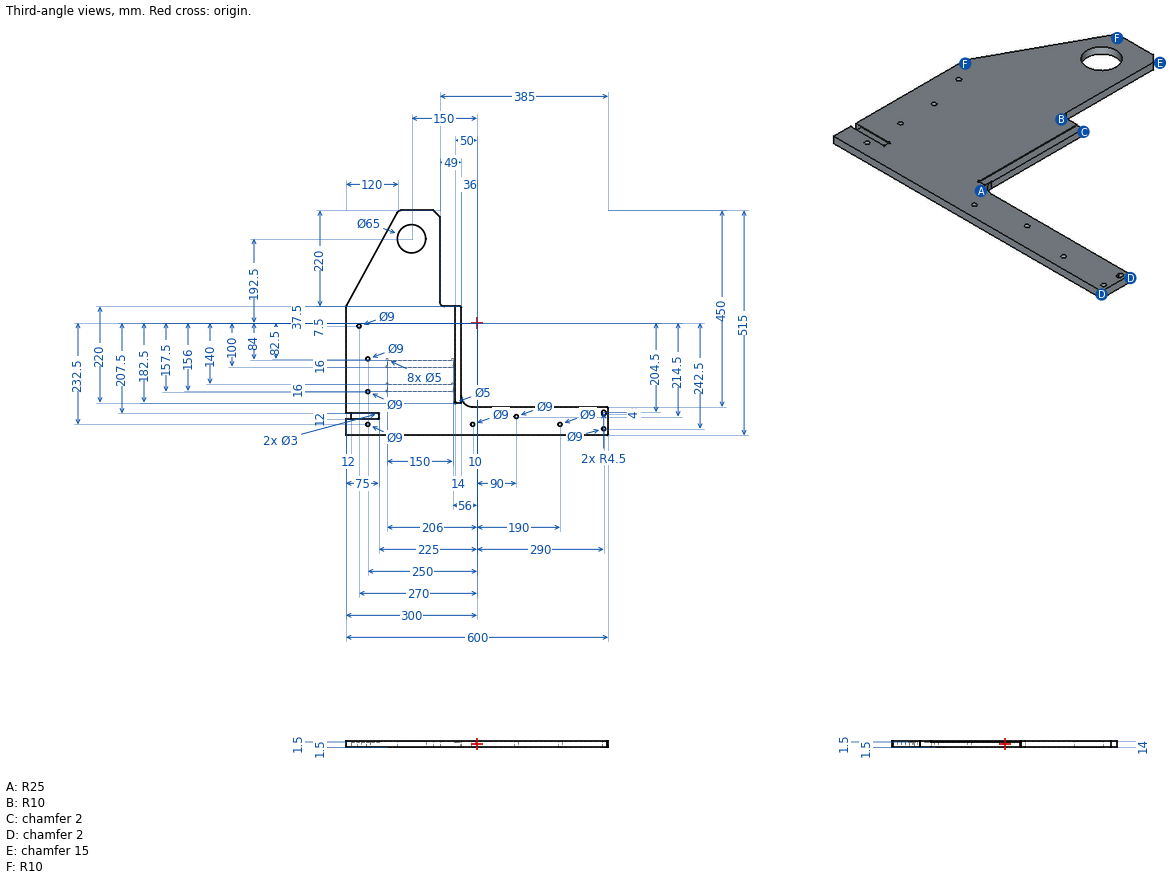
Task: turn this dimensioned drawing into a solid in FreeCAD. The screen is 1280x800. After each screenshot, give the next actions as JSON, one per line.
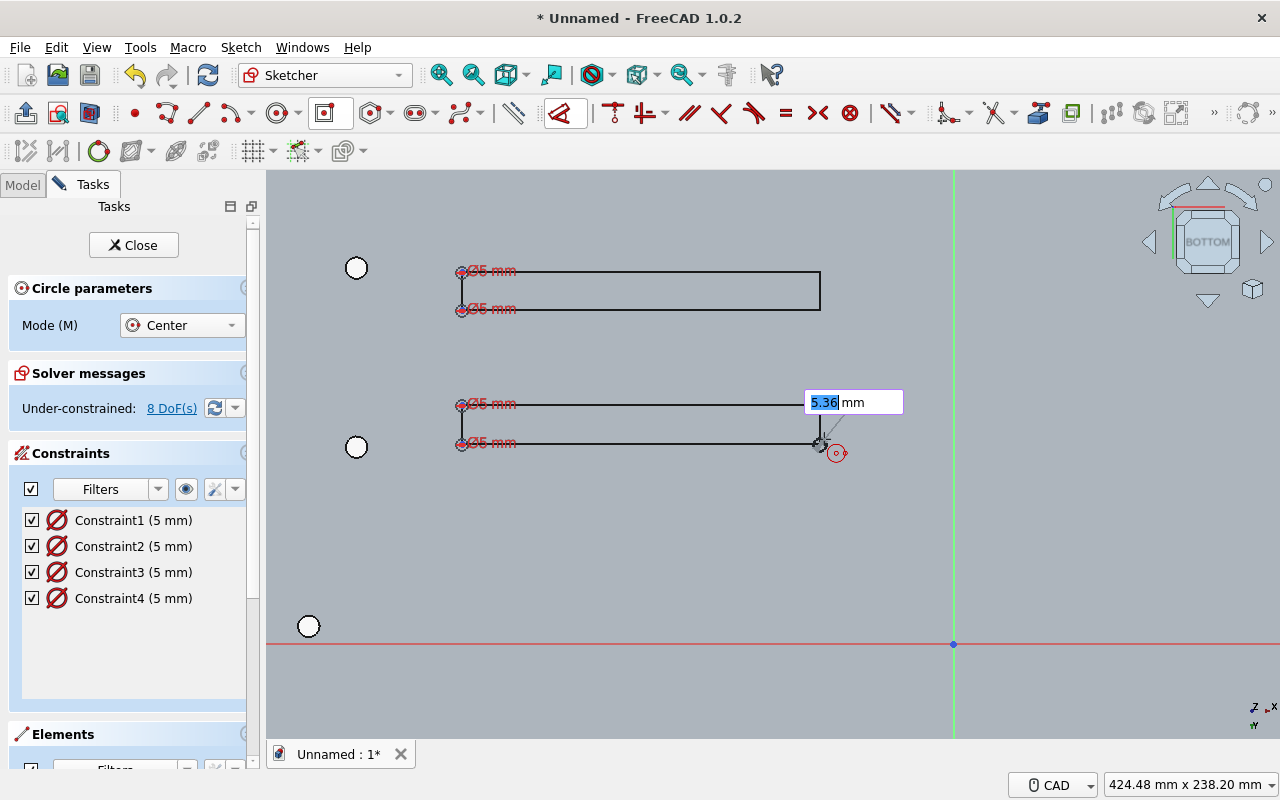
{"action": "type", "text": "5"}
{"action": "key", "text": "Return"}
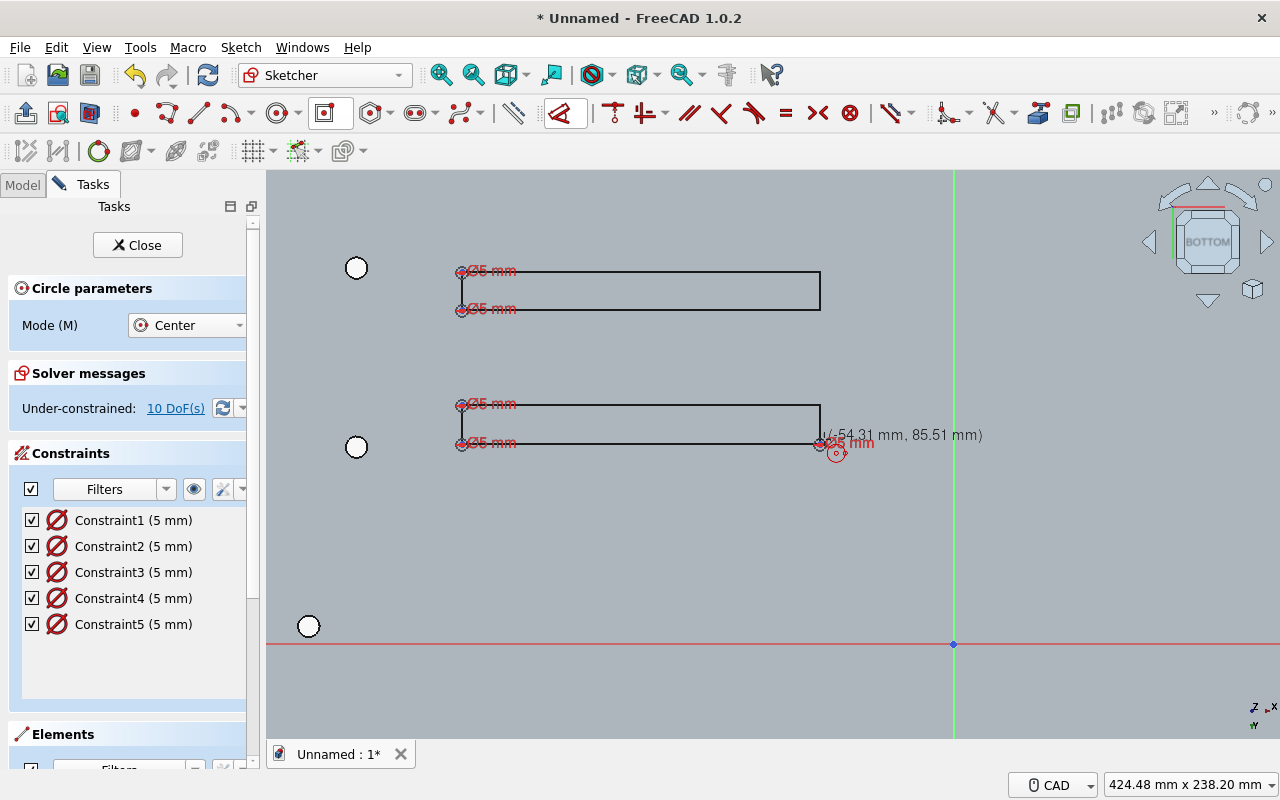
{"action": "scroll", "coordinate": [820, 405], "scroll_direction": "up", "scroll_amount": 7}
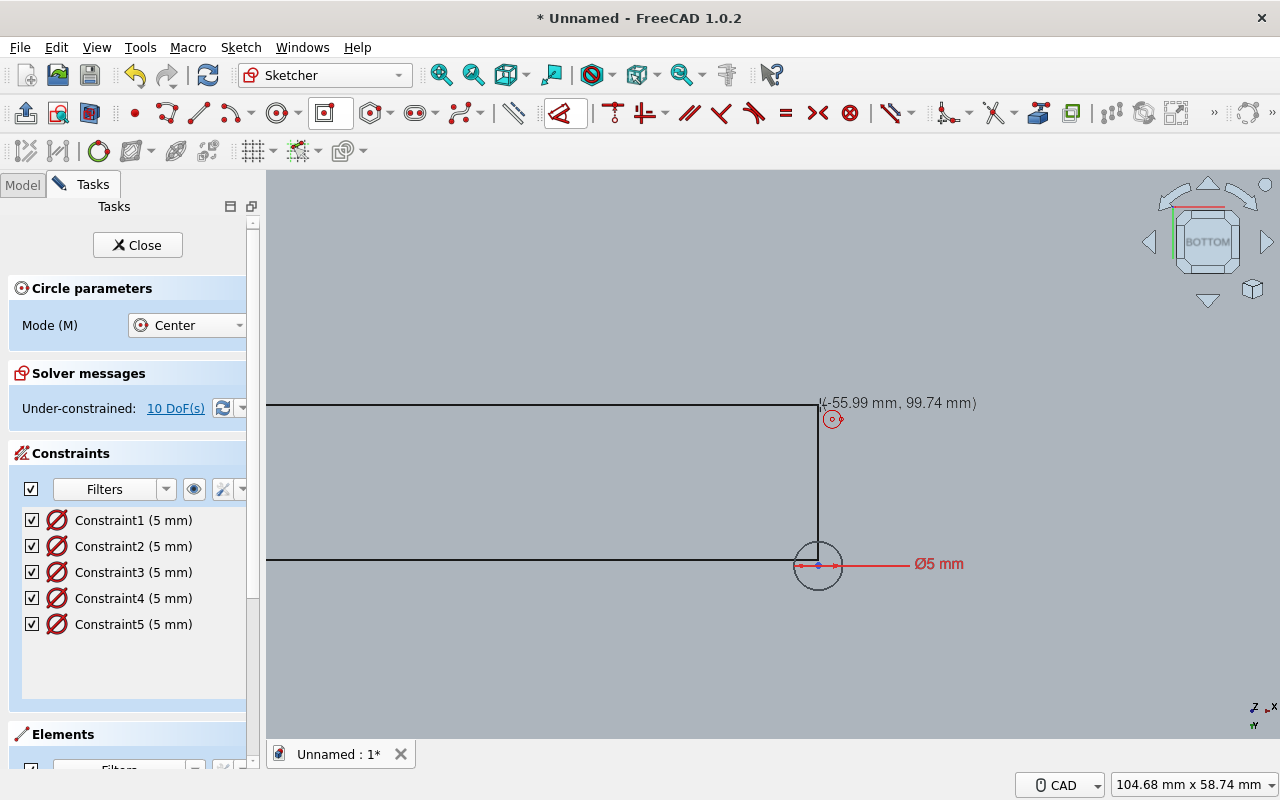
{"action": "scroll", "coordinate": [820, 405], "scroll_direction": "down", "scroll_amount": 7}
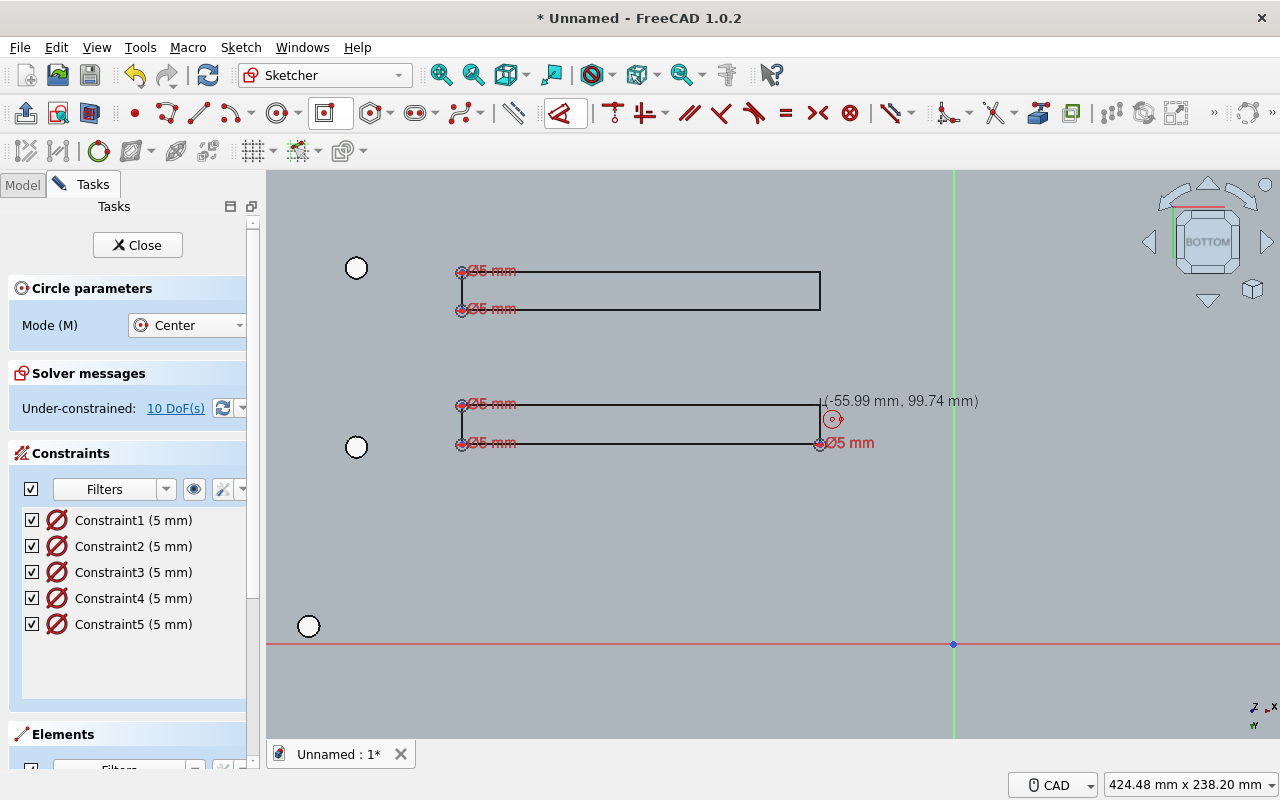
{"action": "left_click", "coordinate": [820, 405]}
{"action": "mouse_move", "coordinate": [824, 401]}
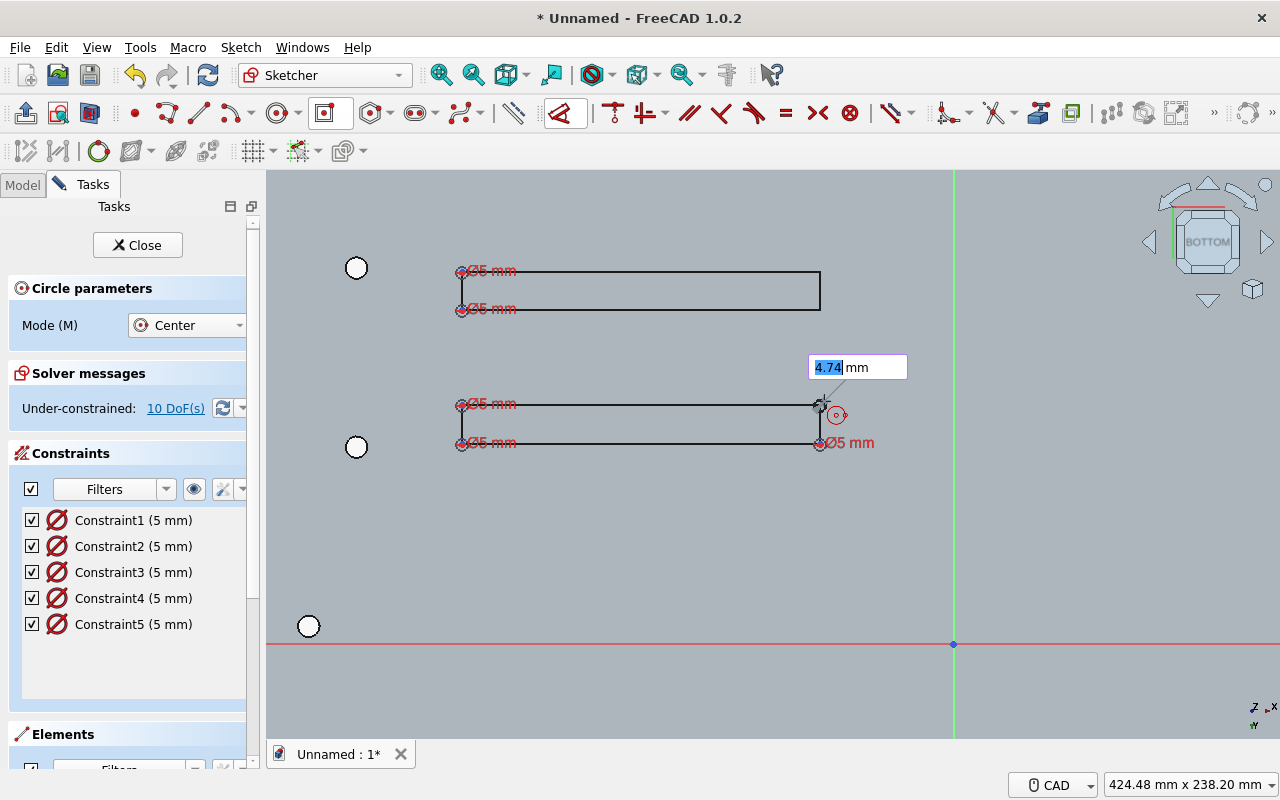
{"action": "type", "text": "5"}
{"action": "key", "text": "Return"}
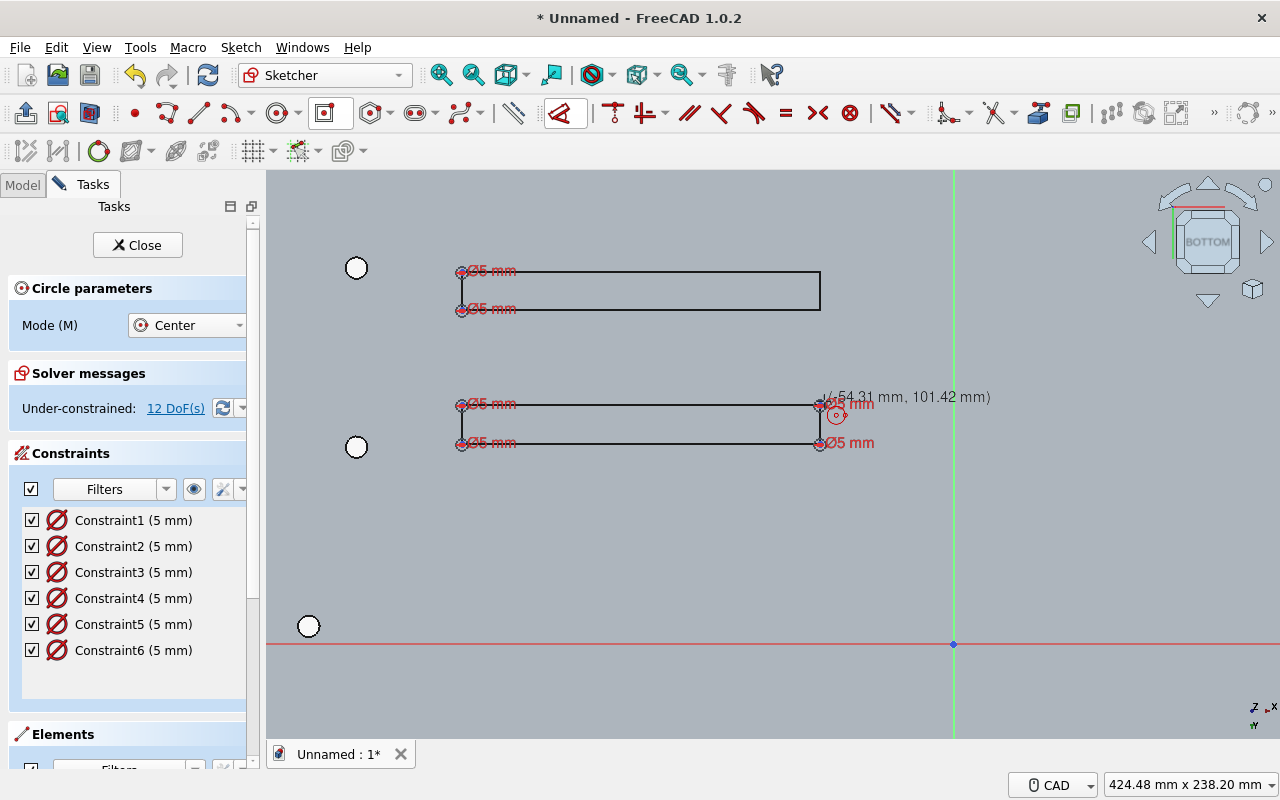
{"action": "scroll", "coordinate": [820, 310], "scroll_direction": "up", "scroll_amount": 7}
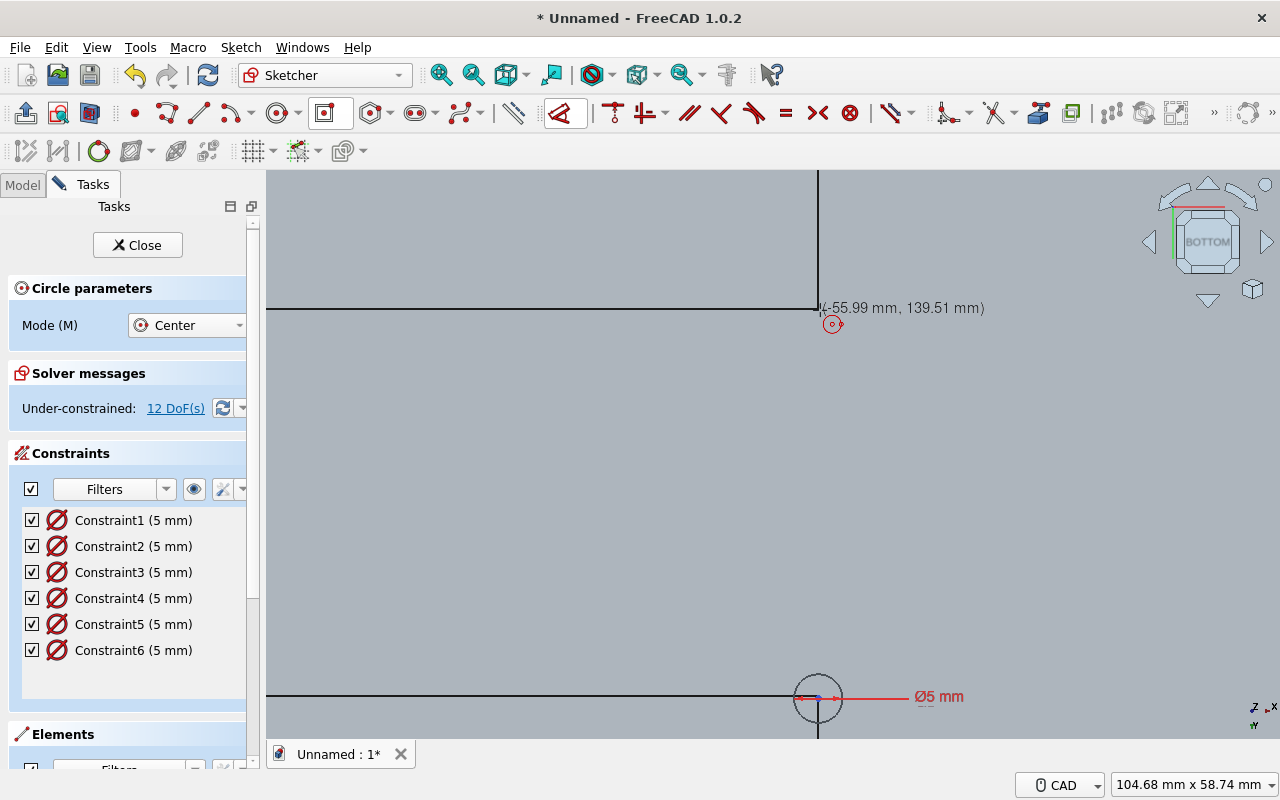
{"action": "scroll", "coordinate": [820, 310], "scroll_direction": "down", "scroll_amount": 7}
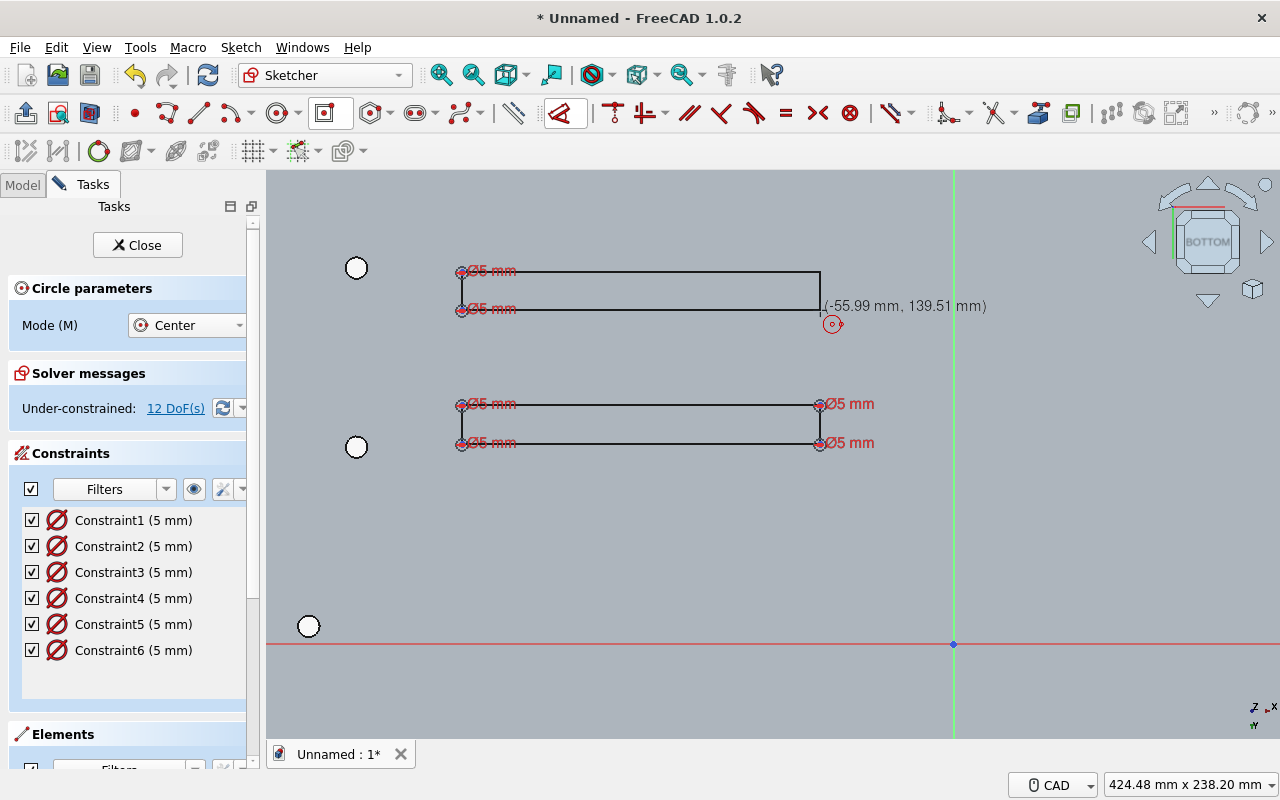
{"action": "left_click", "coordinate": [820, 310]}
{"action": "mouse_move", "coordinate": [824, 306]}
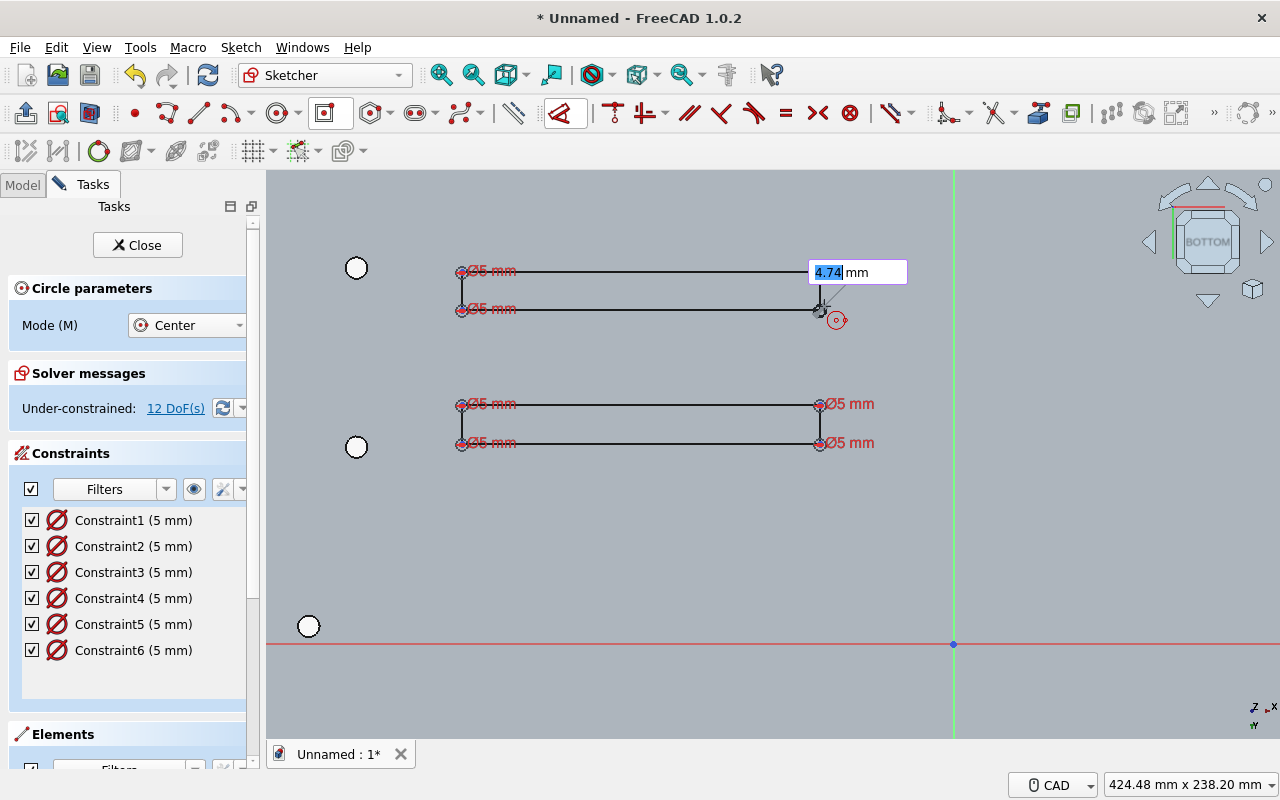
{"action": "type", "text": "5"}
{"action": "key", "text": "Return"}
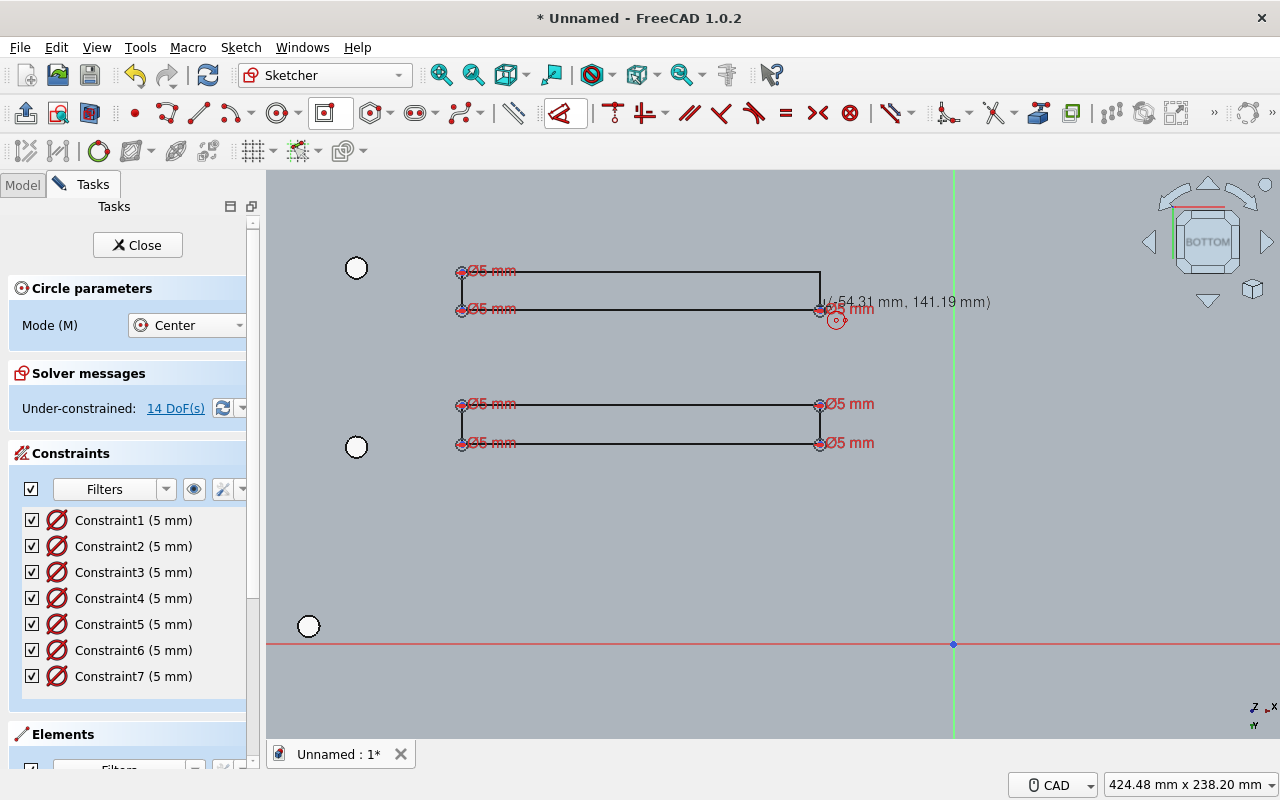
{"action": "scroll", "coordinate": [820, 272], "scroll_direction": "up", "scroll_amount": 7}